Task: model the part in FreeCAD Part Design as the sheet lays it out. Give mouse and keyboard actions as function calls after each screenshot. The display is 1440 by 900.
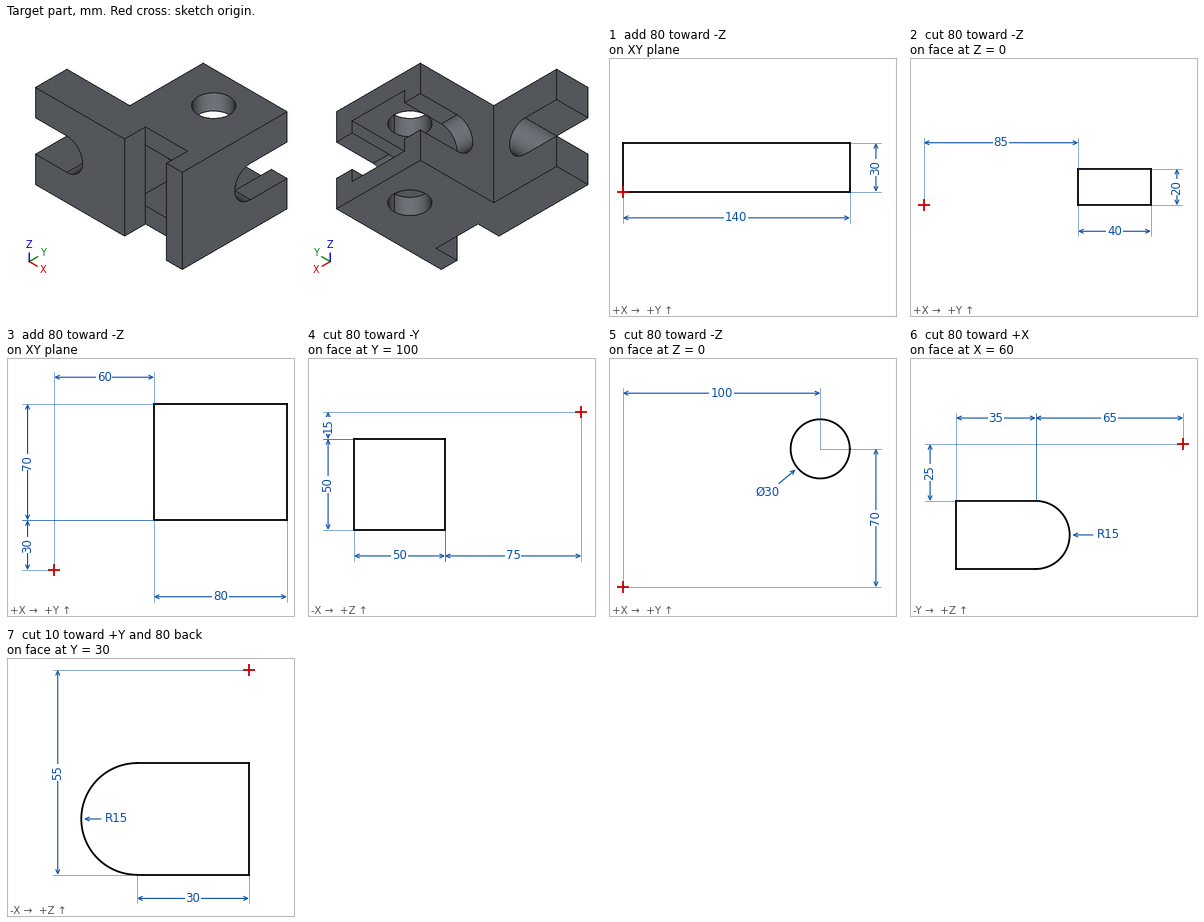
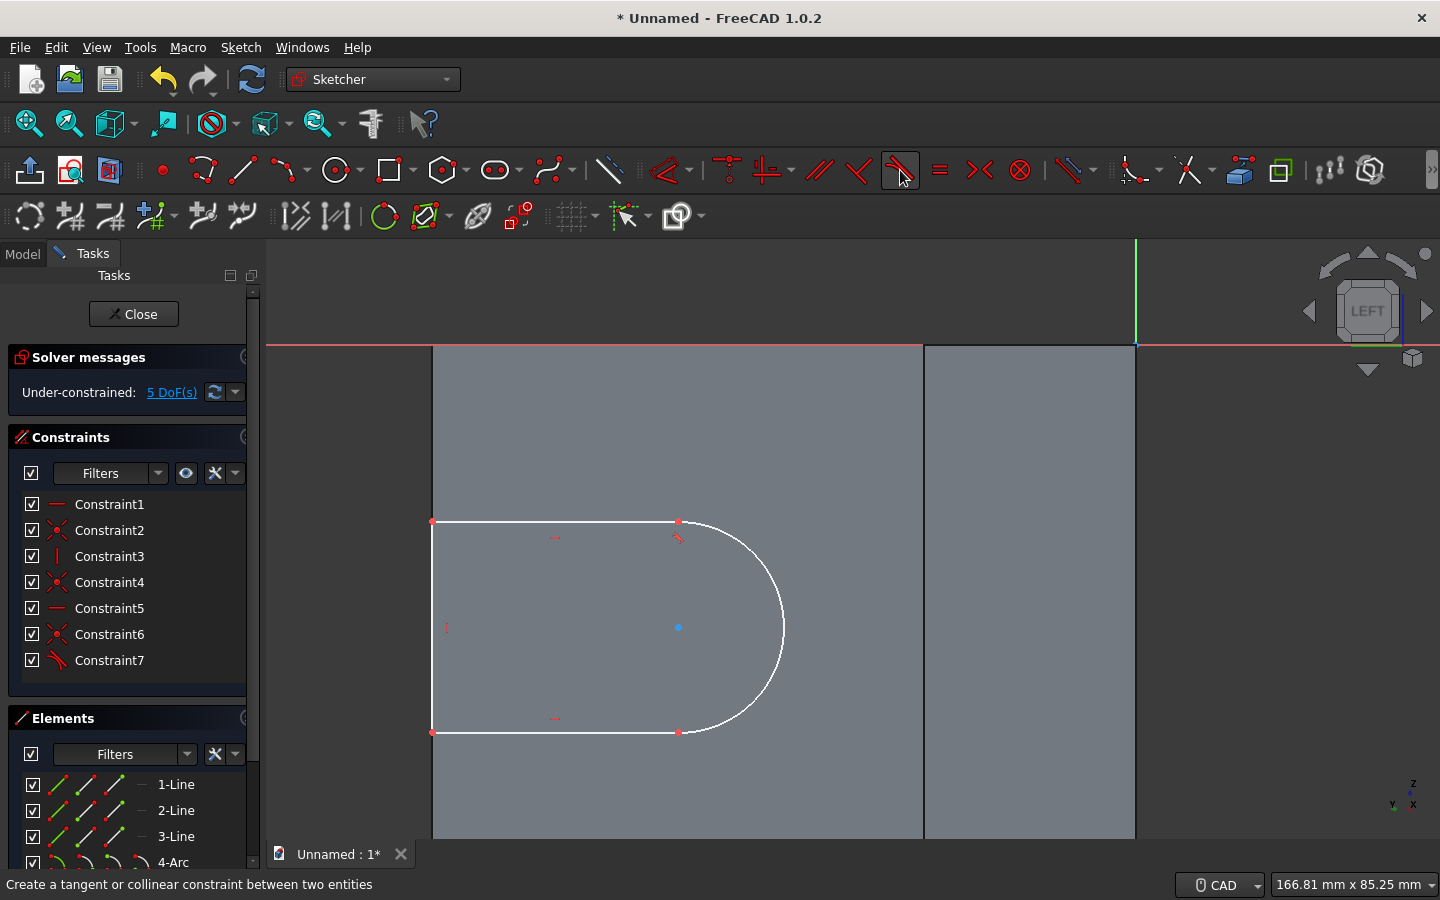
click(506, 733)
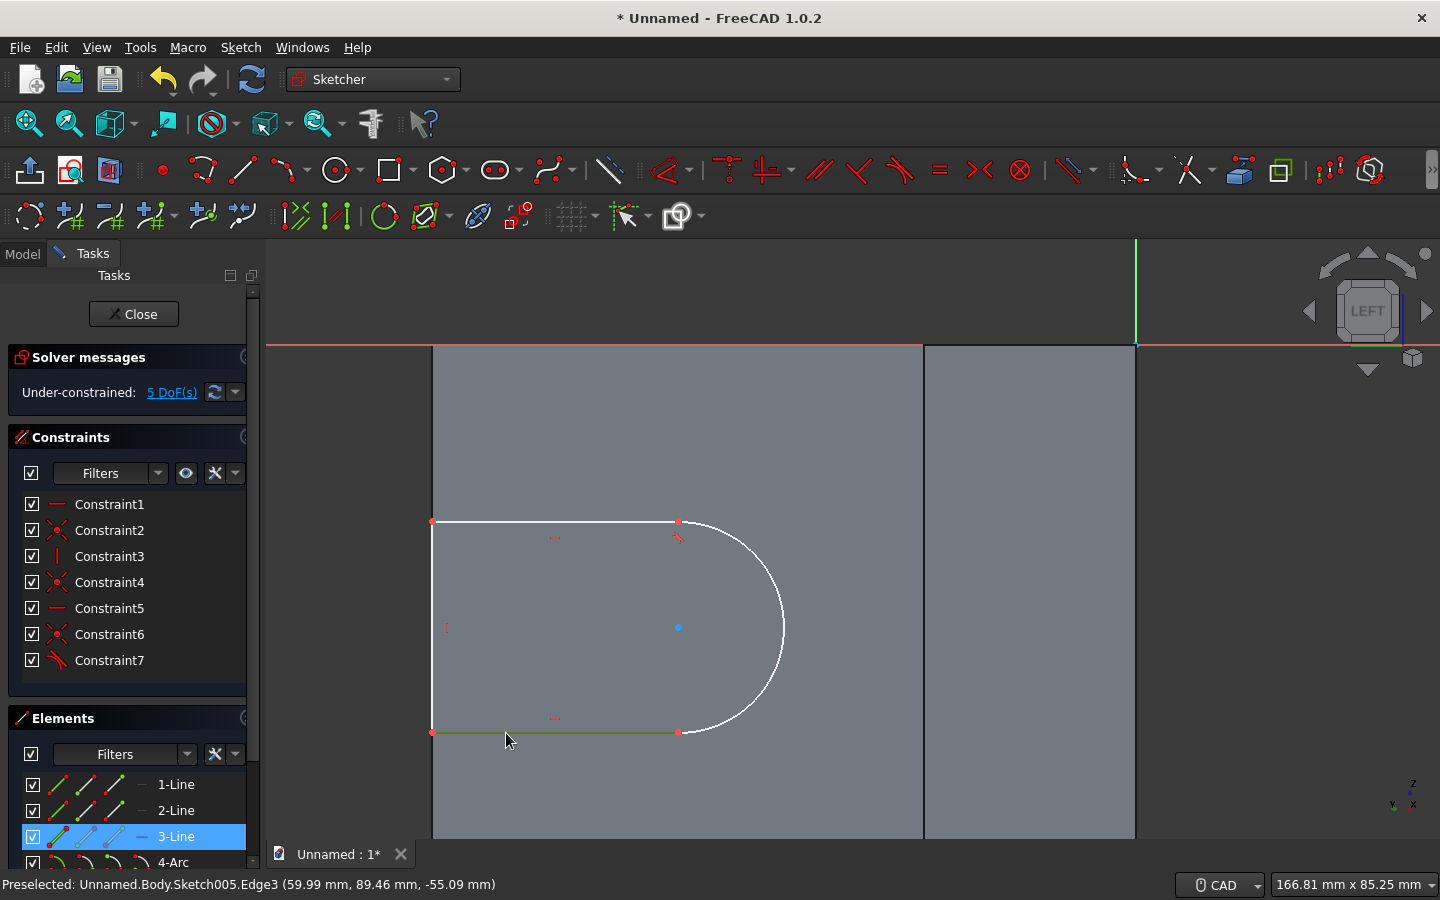
click(764, 690)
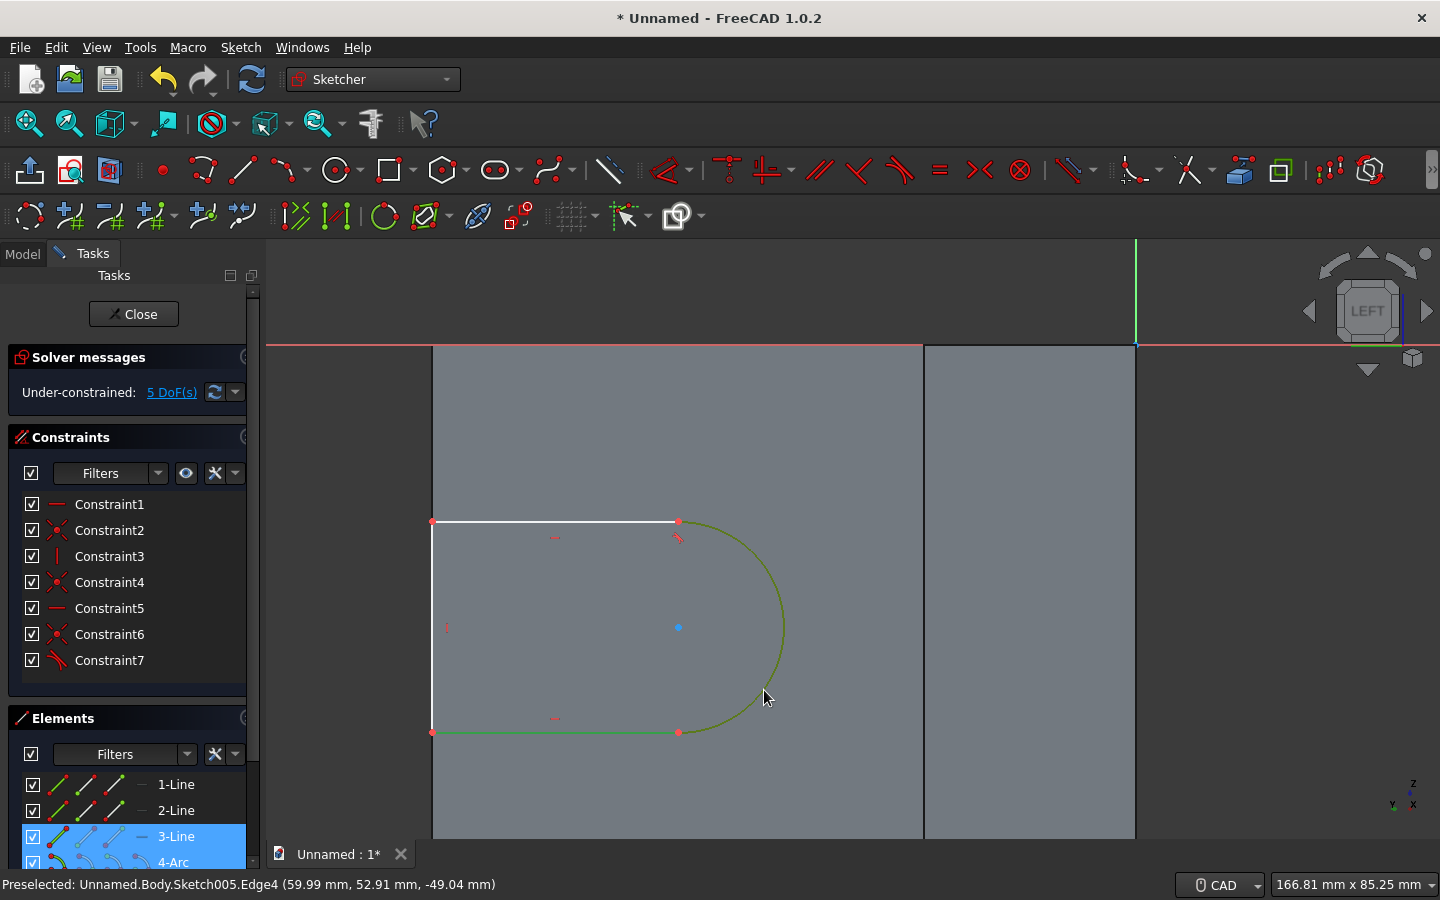
key(t)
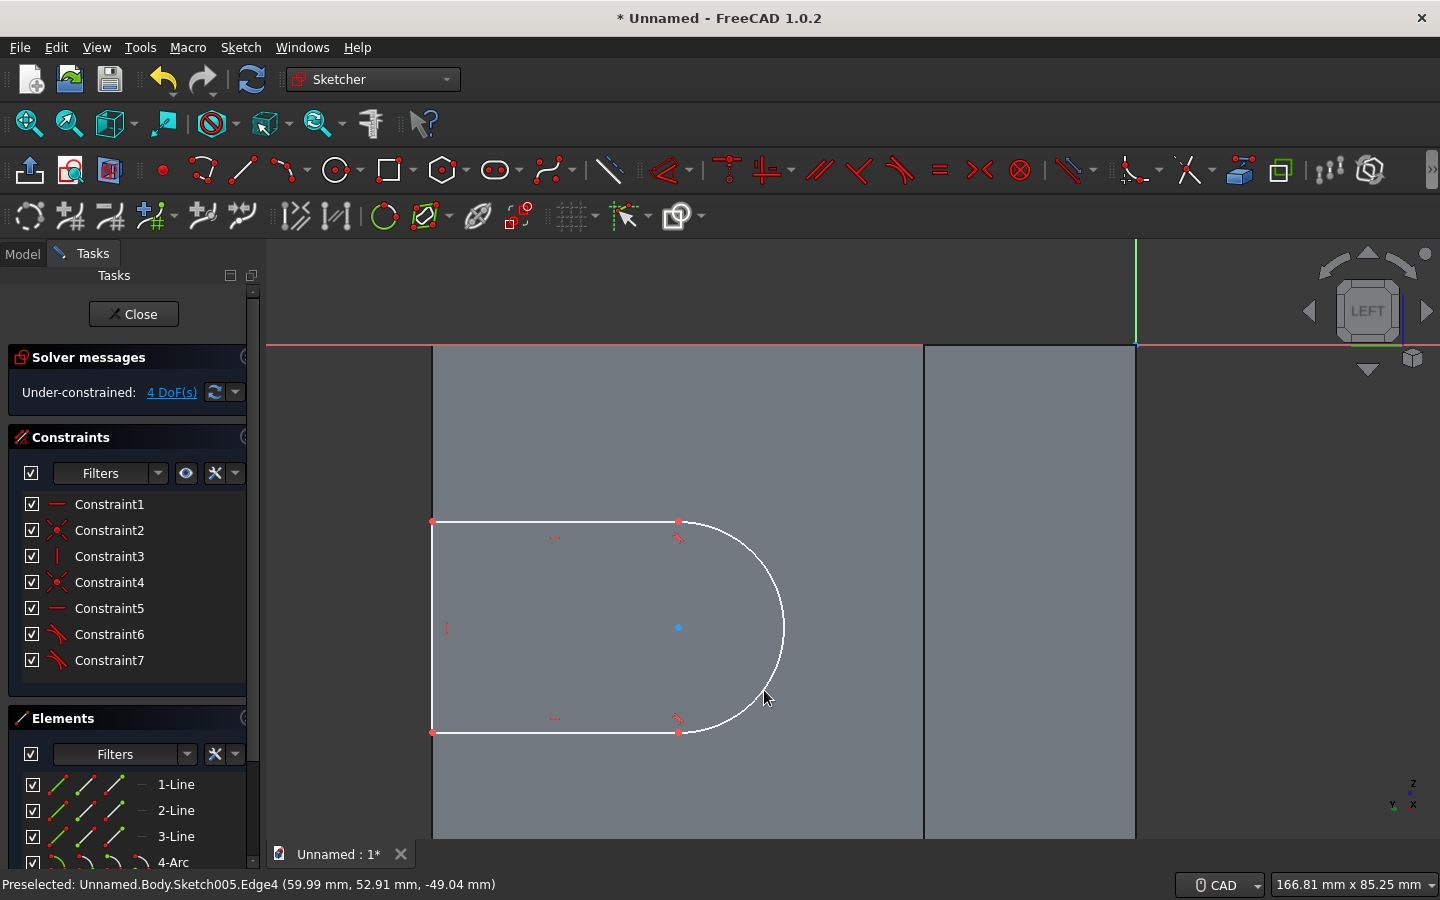
key(d)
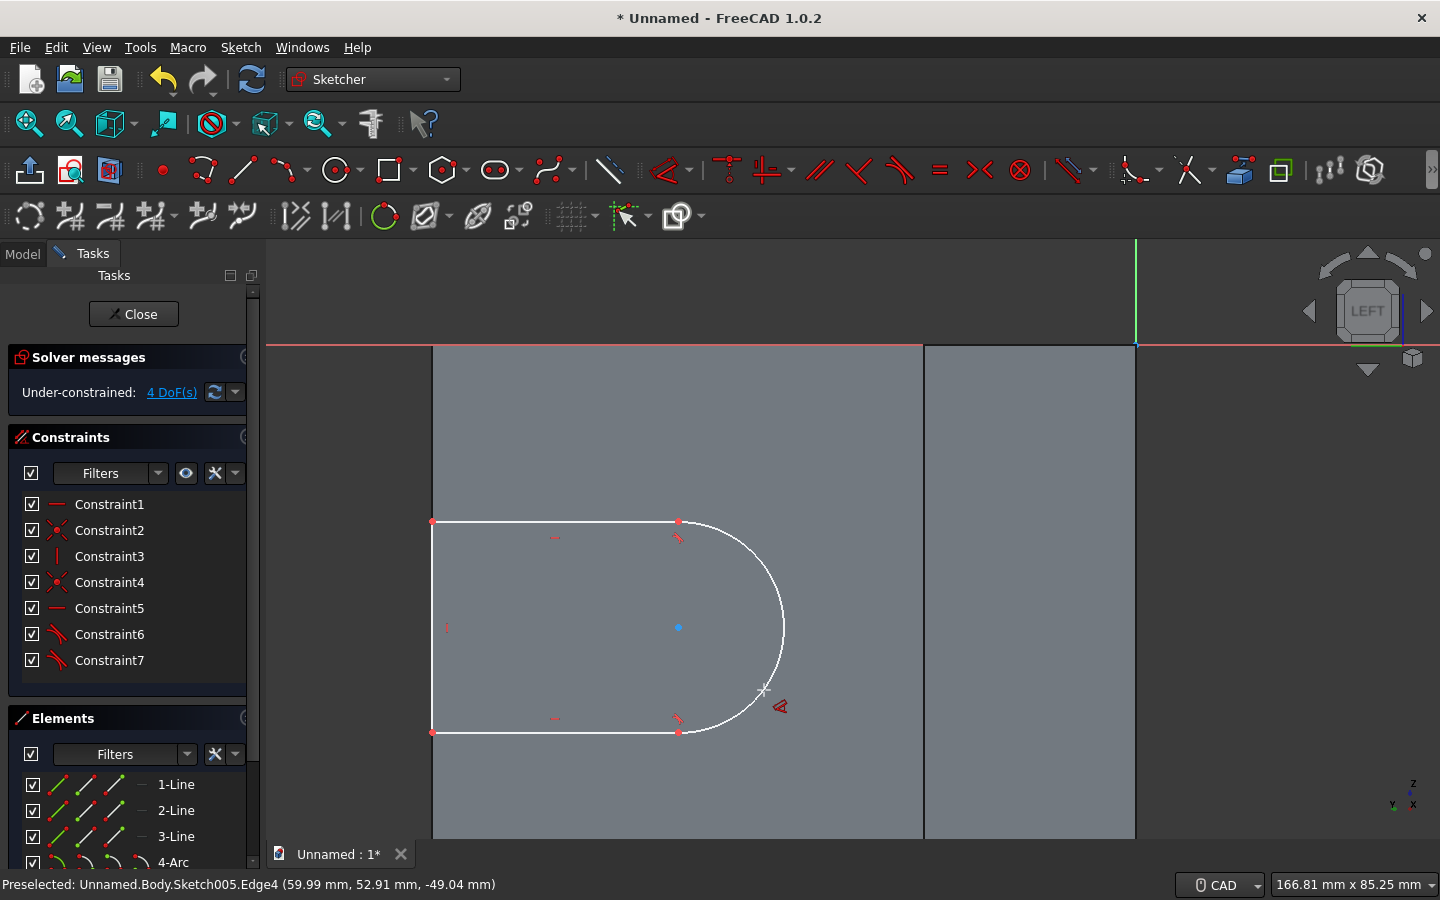
click(764, 690)
click(790, 709)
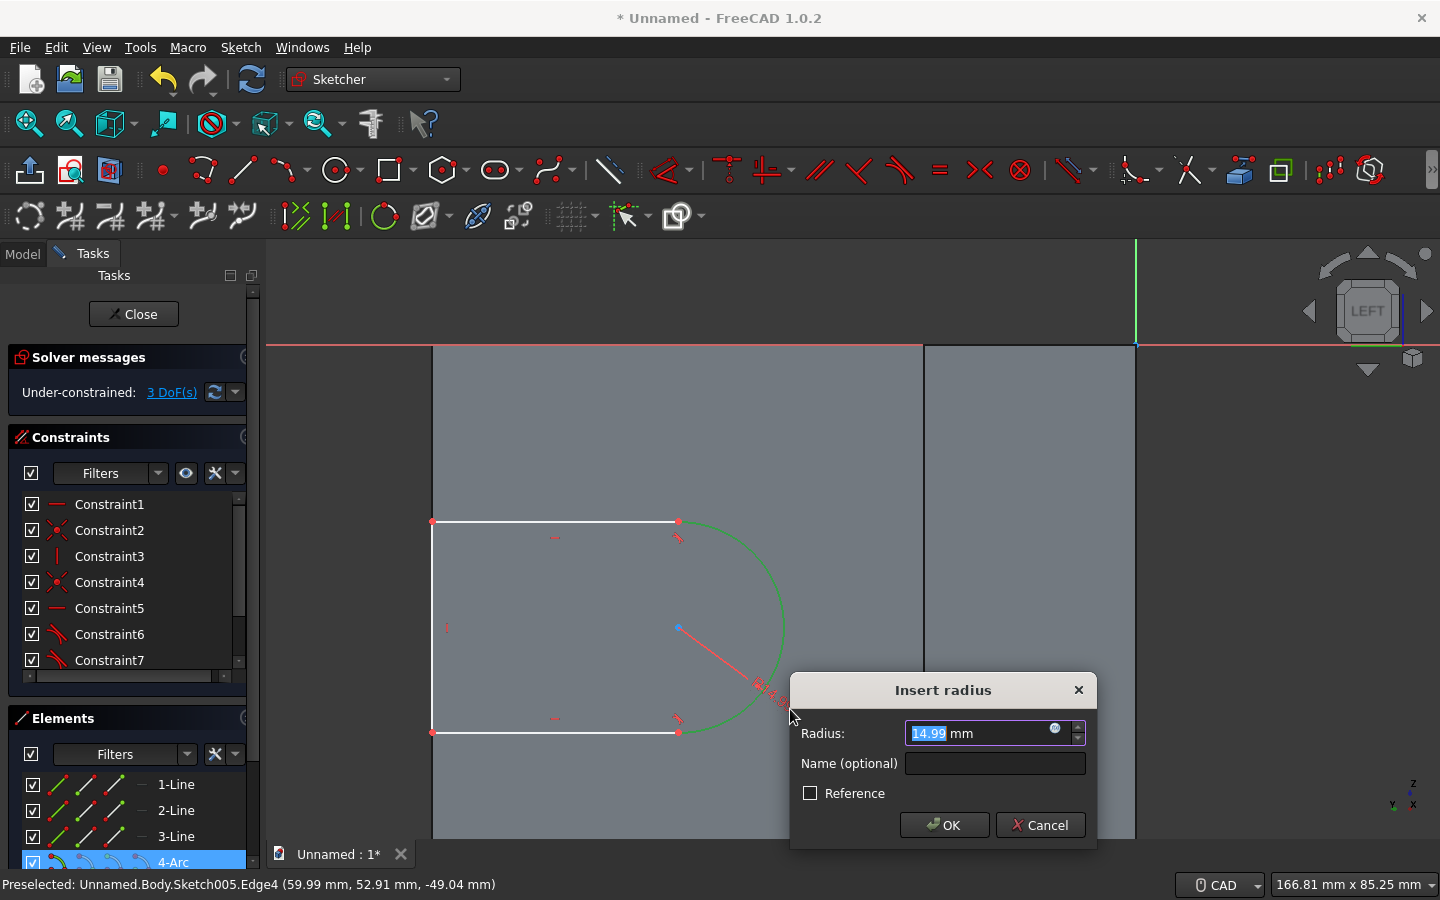
text(15)
key(Return)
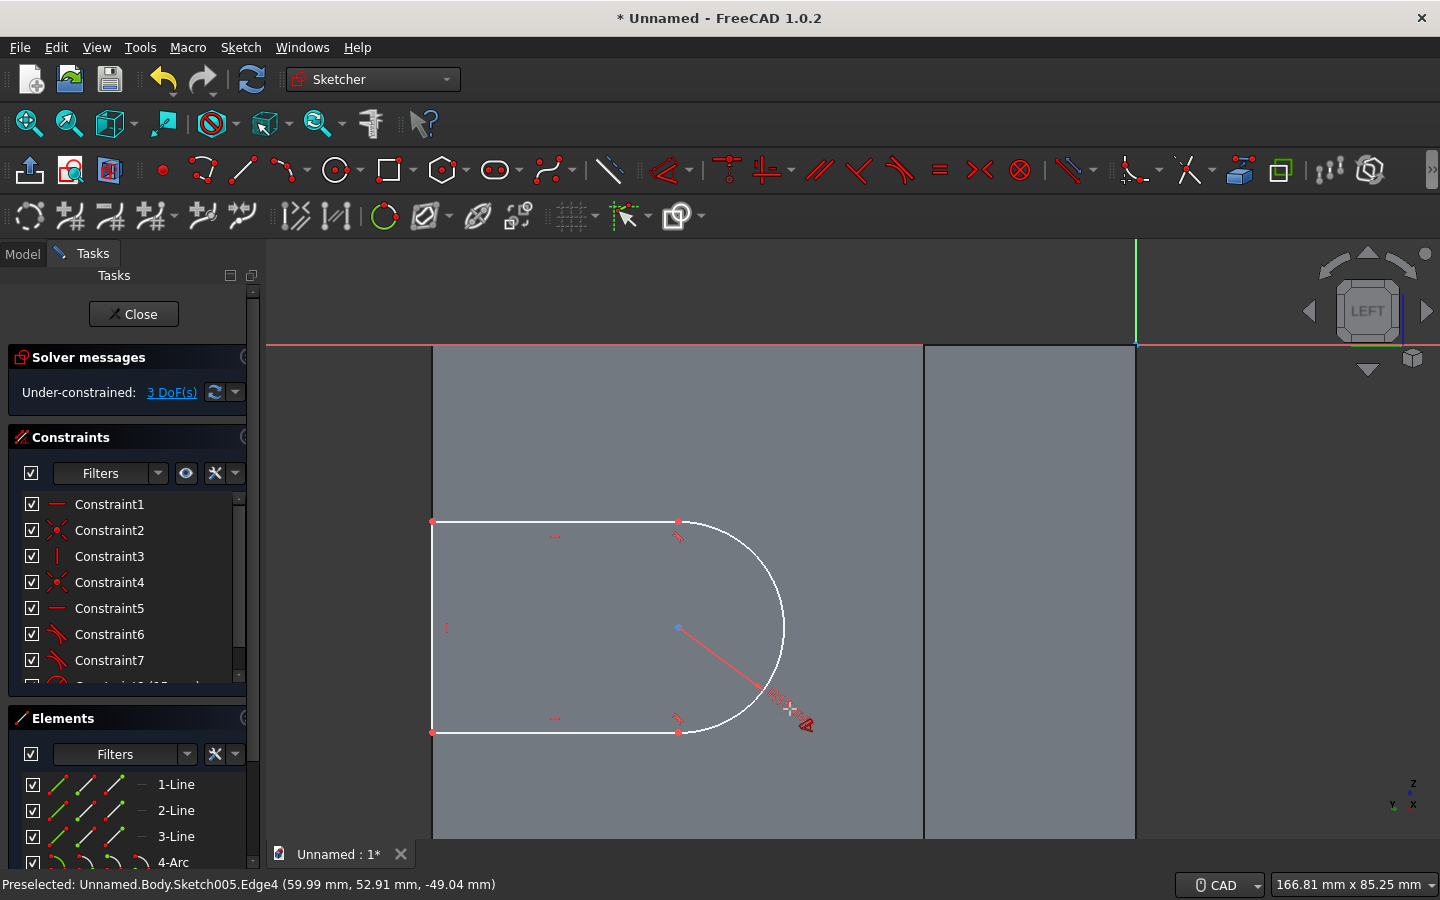
click(605, 522)
click(555, 488)